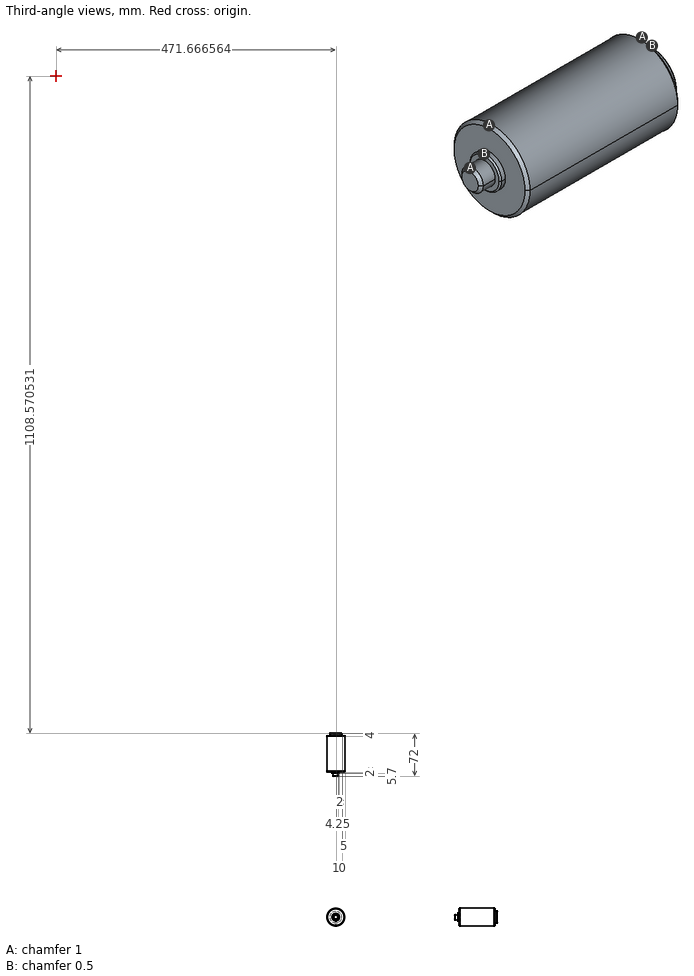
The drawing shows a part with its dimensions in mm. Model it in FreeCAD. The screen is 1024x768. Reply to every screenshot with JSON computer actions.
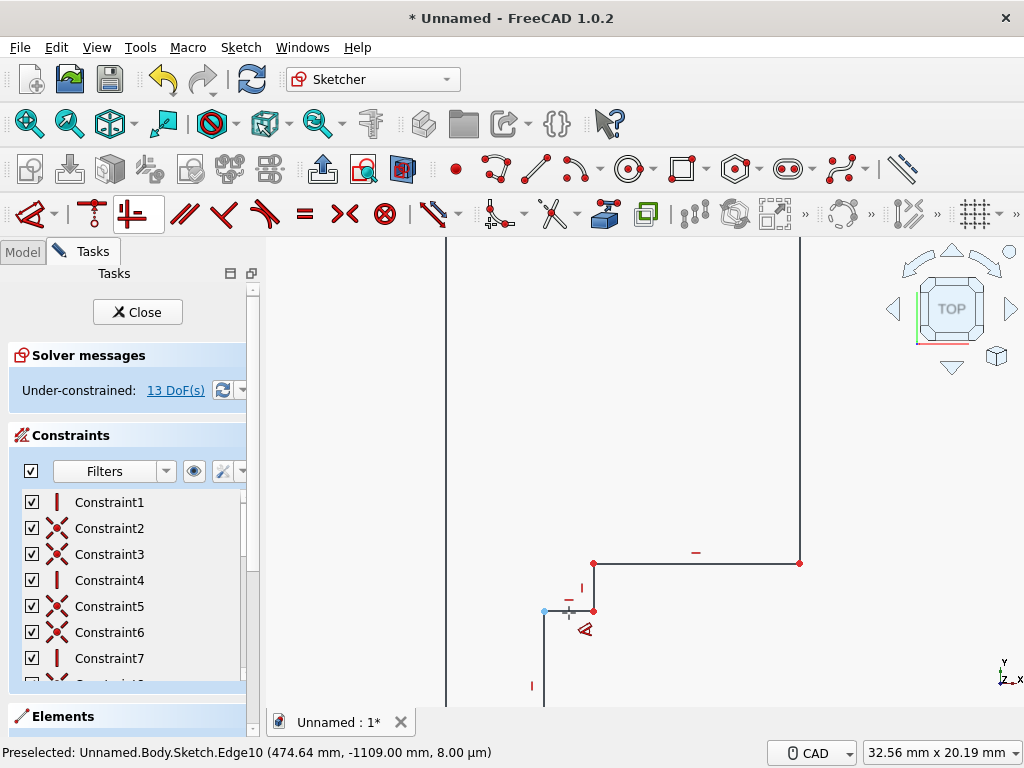
{"action": "left_click", "coordinate": [569, 611]}
{"action": "left_click", "coordinate": [569, 645]}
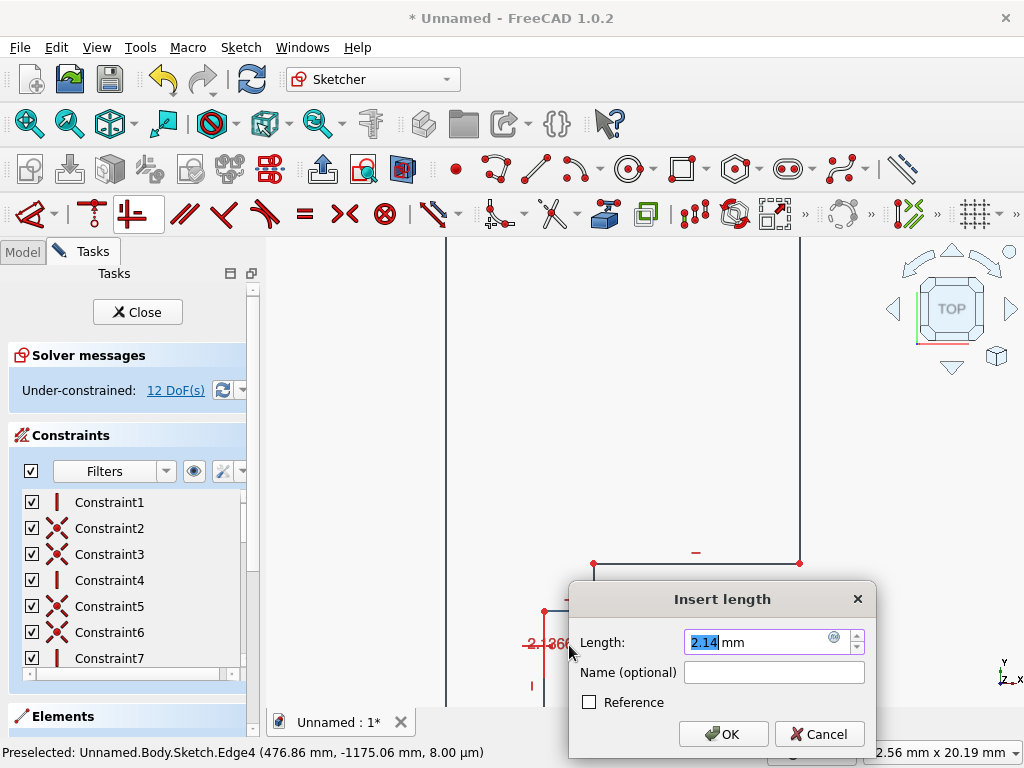
{"action": "type", "text": "2"}
{"action": "key", "text": "Return"}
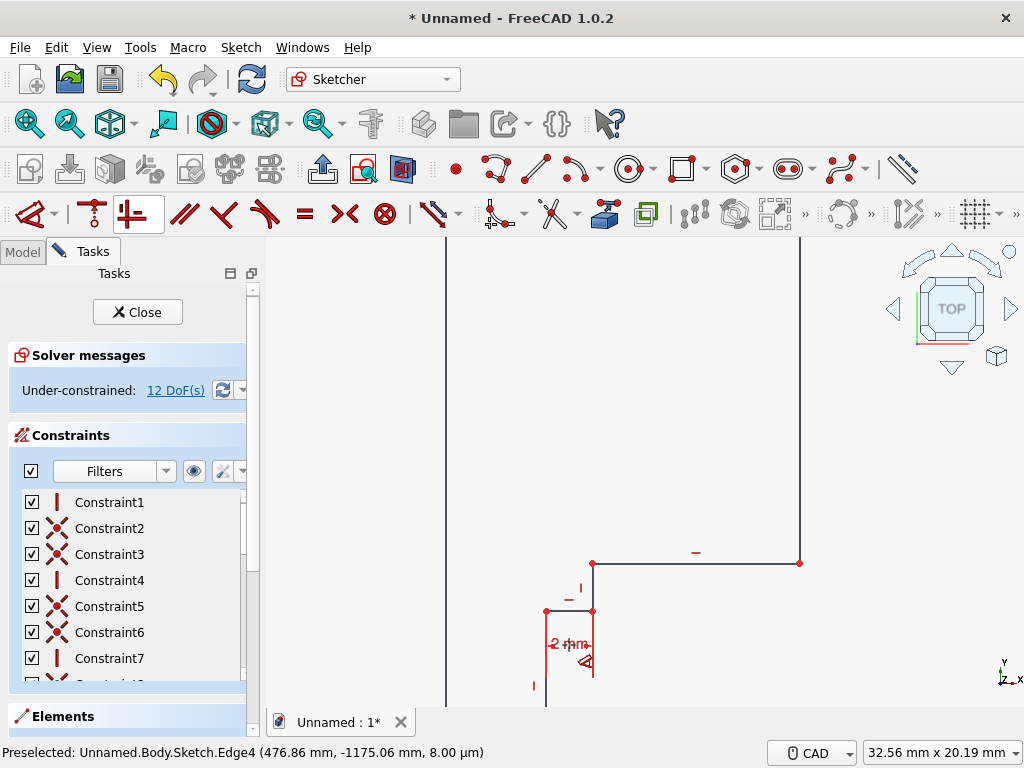
{"action": "left_click", "coordinate": [593, 597]}
{"action": "left_click", "coordinate": [559, 588]}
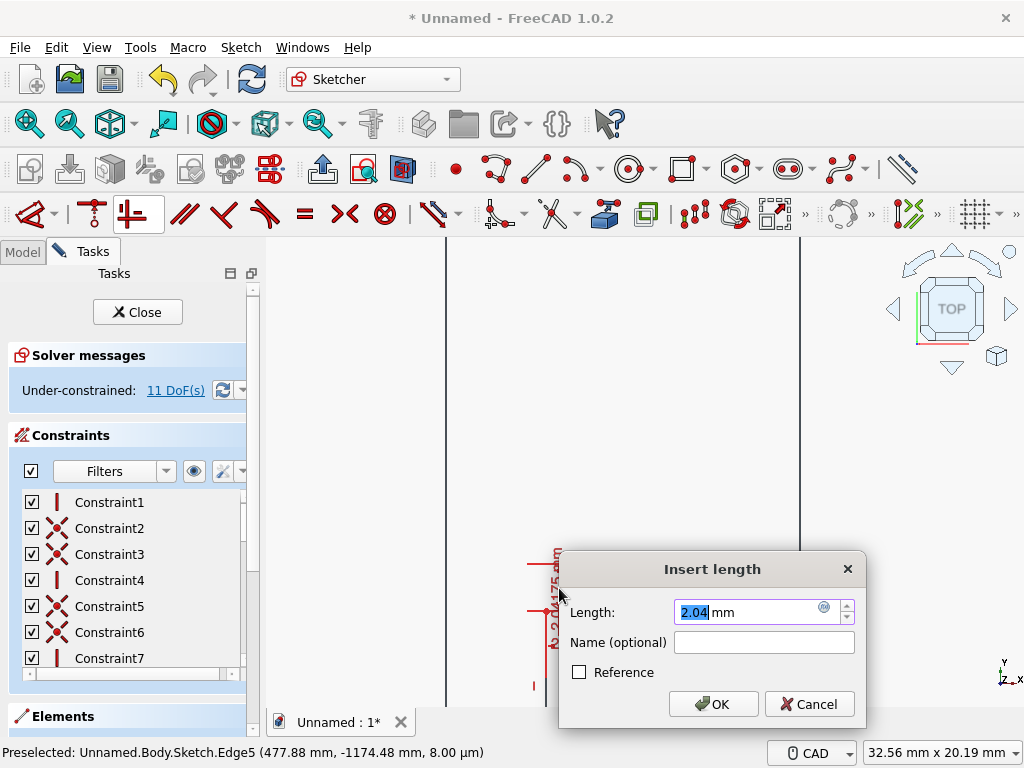
{"action": "type", "text": "2"}
{"action": "key", "text": "Return"}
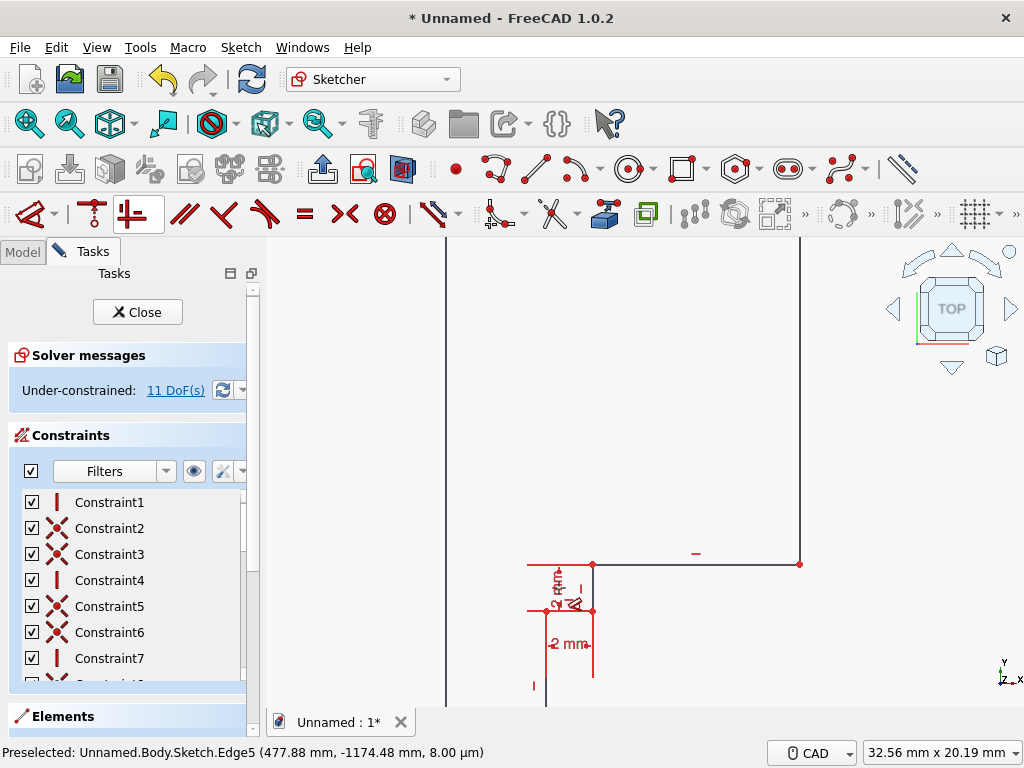
{"action": "scroll", "coordinate": [569, 614], "scroll_direction": "down", "scroll_amount": 10}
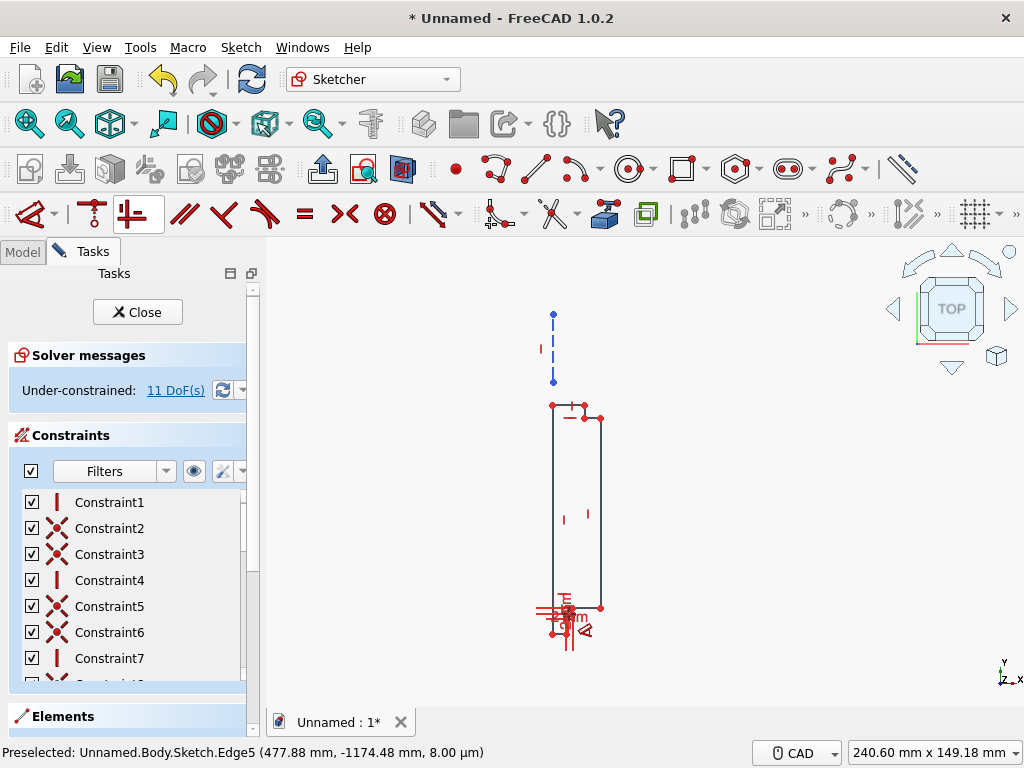
{"action": "scroll", "coordinate": [596, 418], "scroll_direction": "up", "scroll_amount": 6}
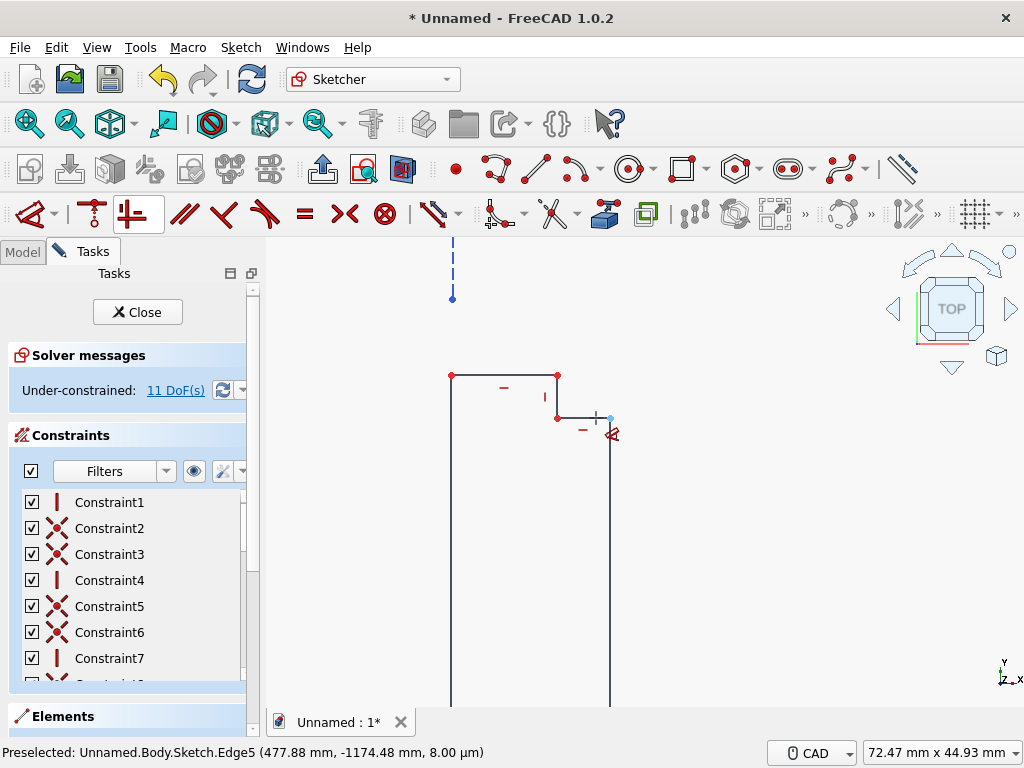
{"action": "left_click", "coordinate": [594, 418]}
{"action": "left_click", "coordinate": [584, 384]}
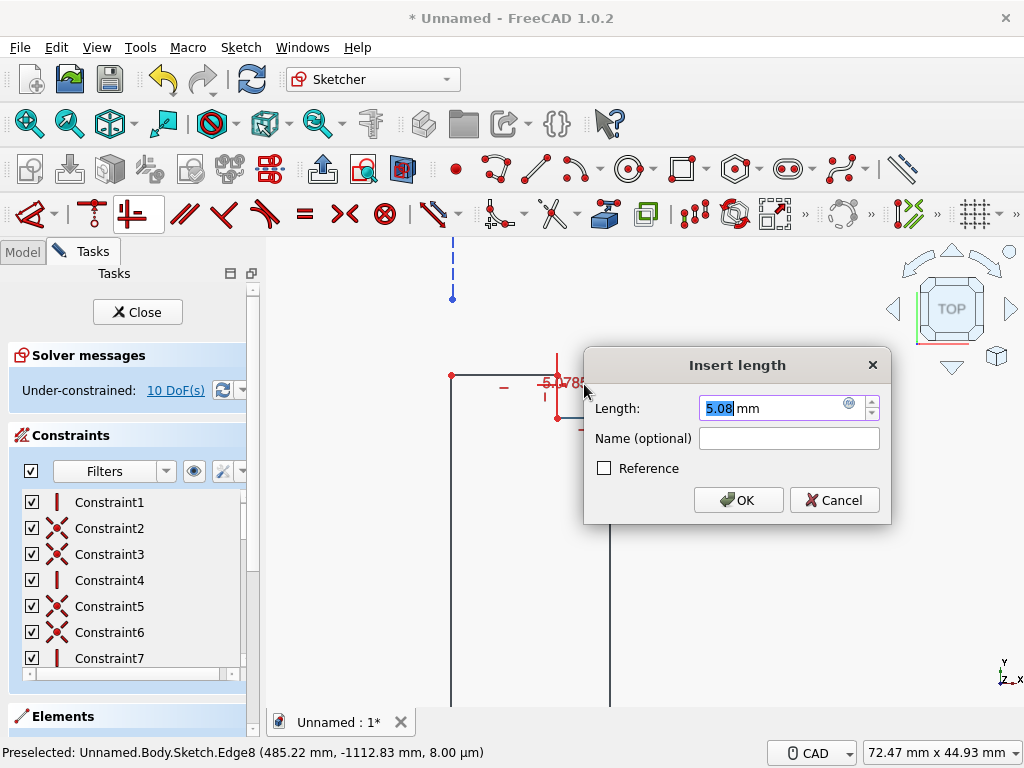
{"action": "type", "text": "5"}
{"action": "key", "text": "Return"}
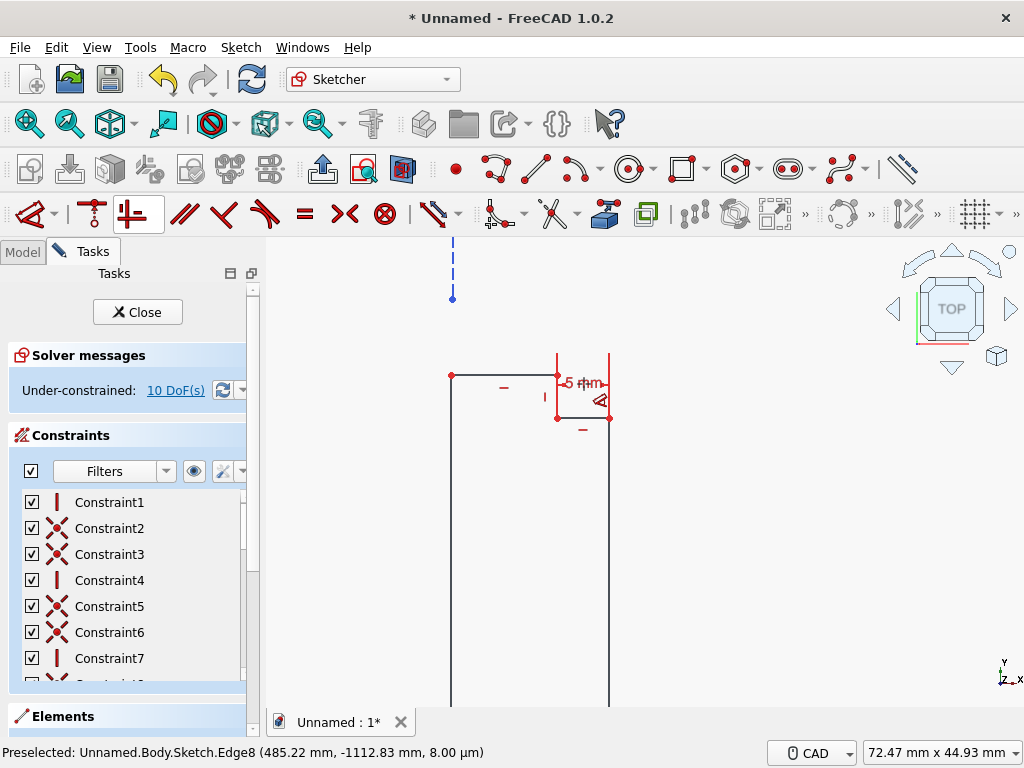
{"action": "left_click", "coordinate": [557, 405]}
{"action": "left_click", "coordinate": [523, 407]}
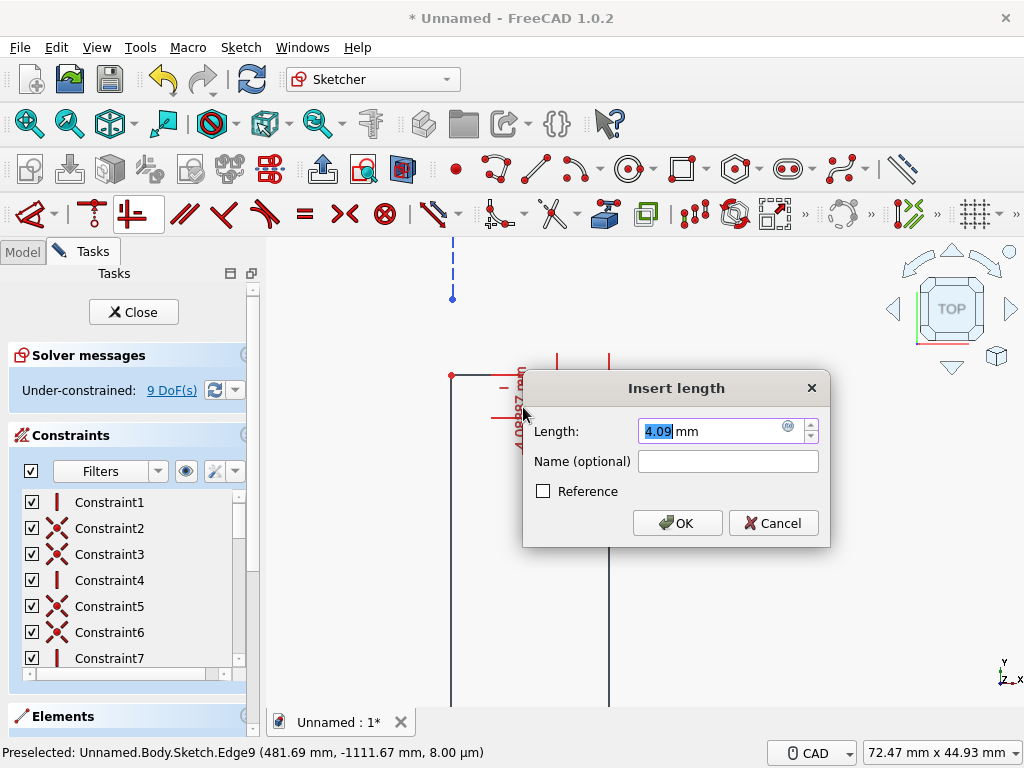
{"action": "type", "text": "4"}
{"action": "key", "text": "Return"}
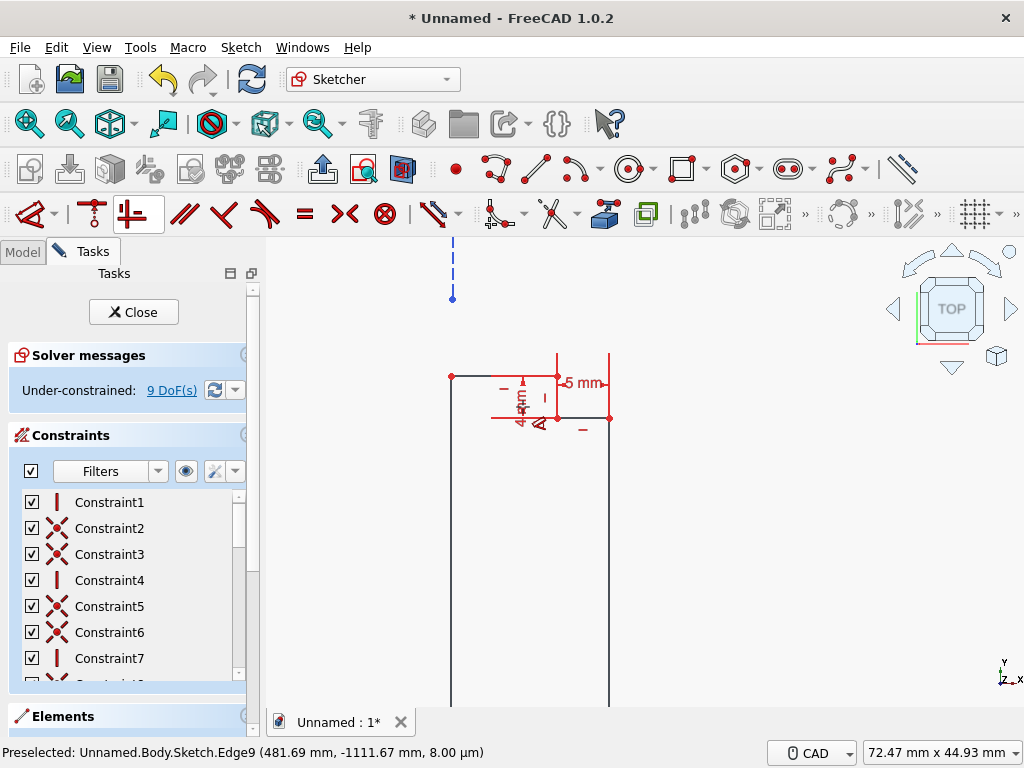
{"action": "scroll", "coordinate": [596, 417], "scroll_direction": "down", "scroll_amount": 6}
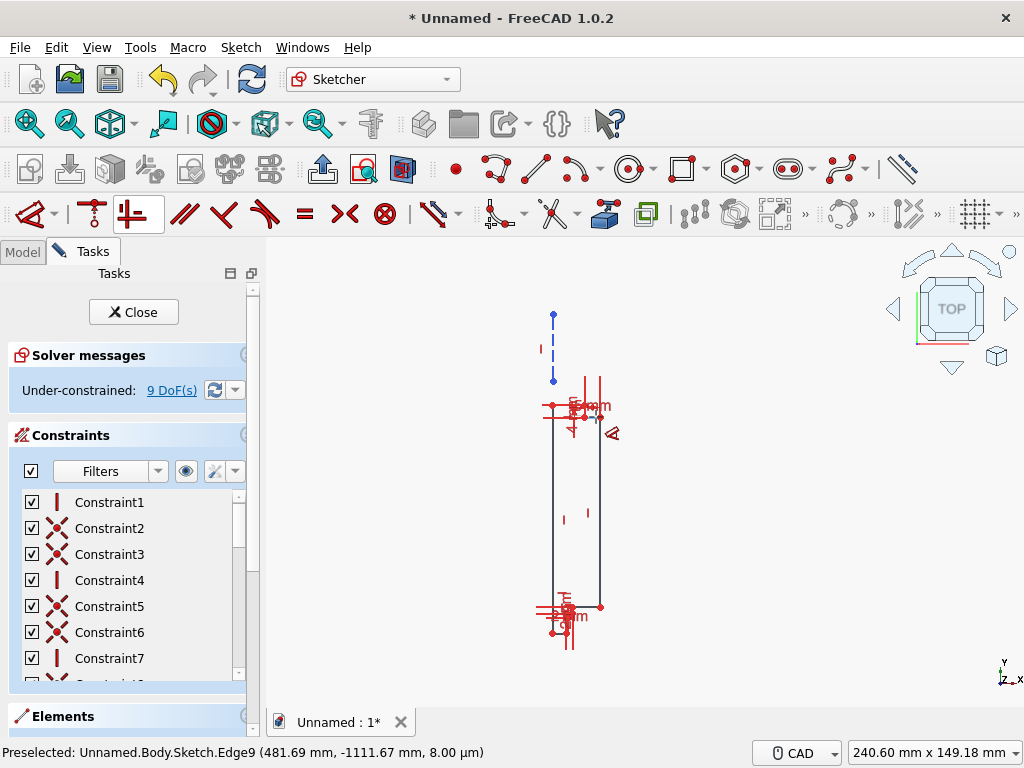
{"action": "left_click", "coordinate": [553, 474]}
{"action": "left_click", "coordinate": [519, 519]}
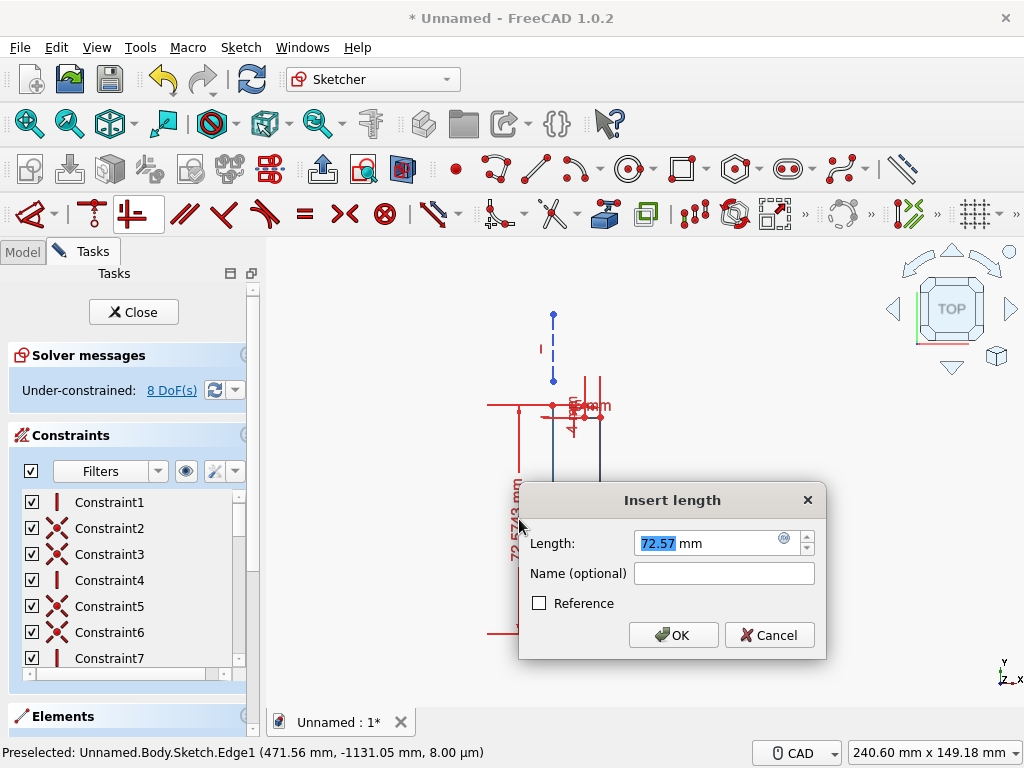
{"action": "type", "text": "72"}
{"action": "key", "text": "Return"}